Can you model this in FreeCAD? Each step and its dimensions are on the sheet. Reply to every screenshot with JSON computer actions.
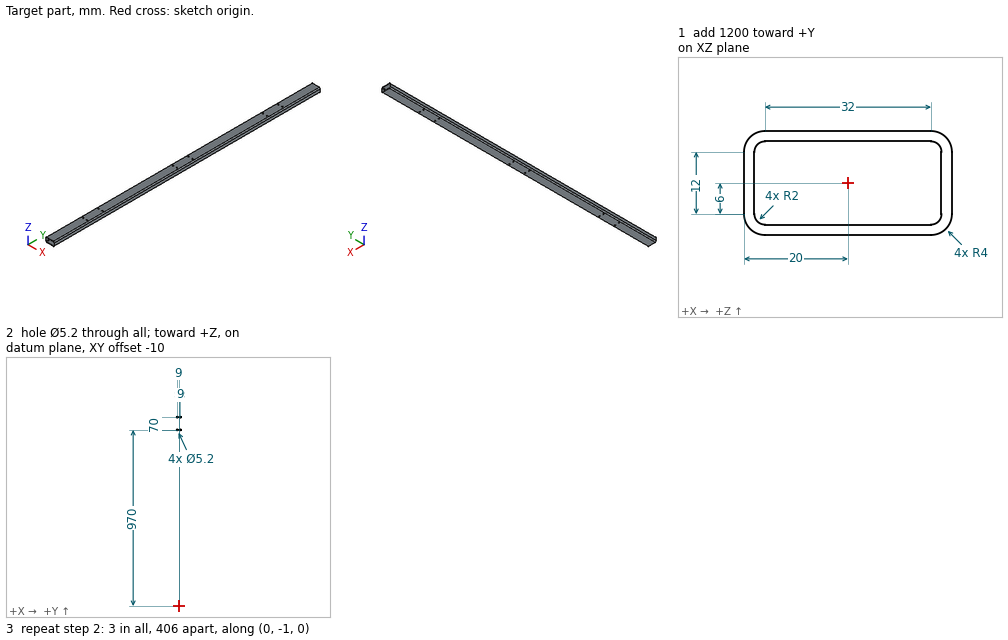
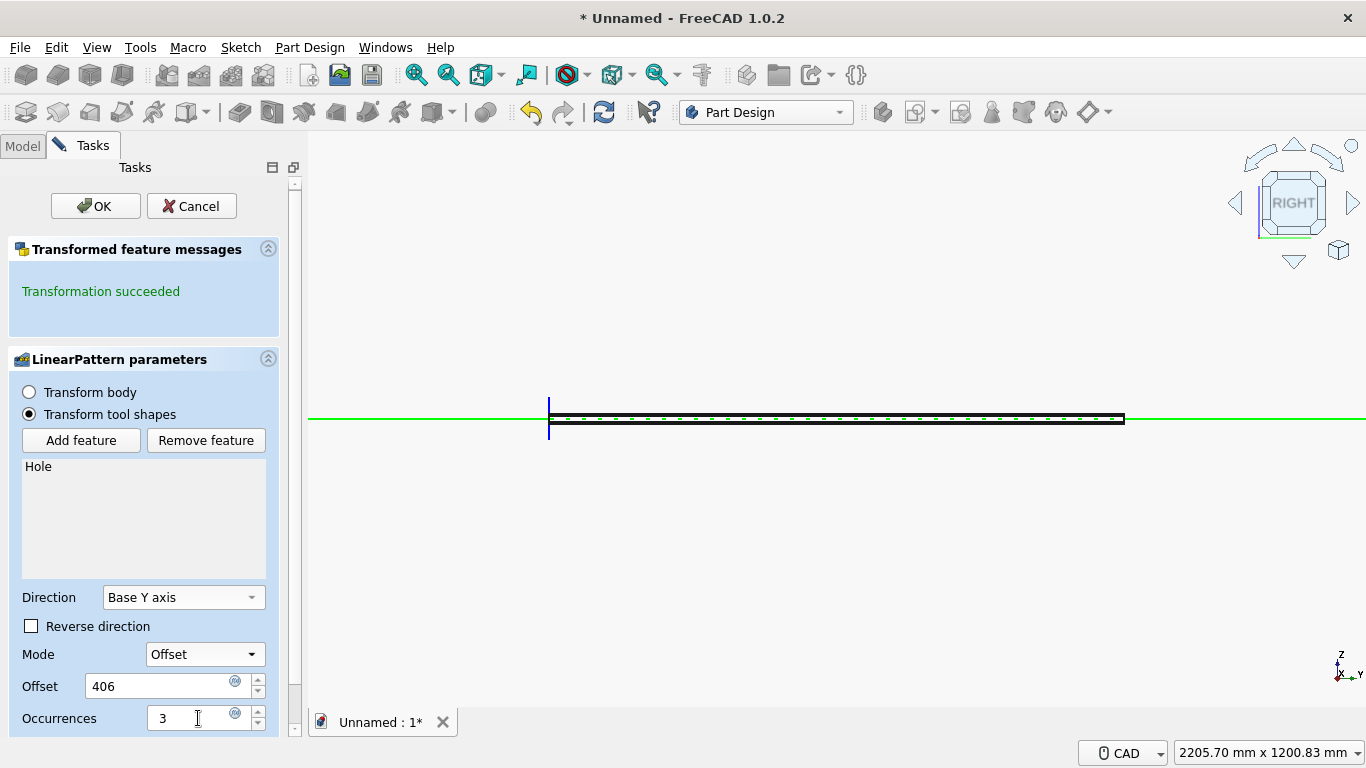
{"action": "left_click", "coordinate": [30, 626]}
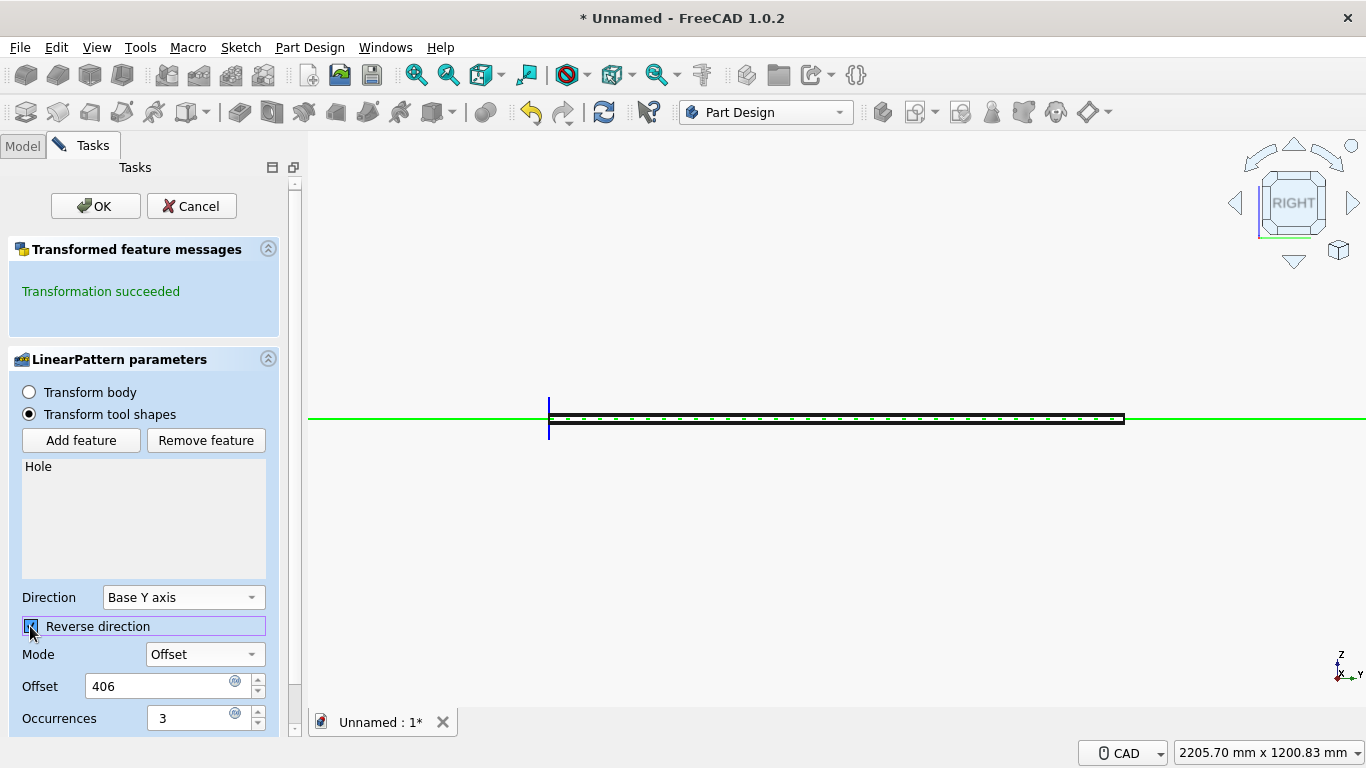
{"action": "left_click", "coordinate": [96, 206]}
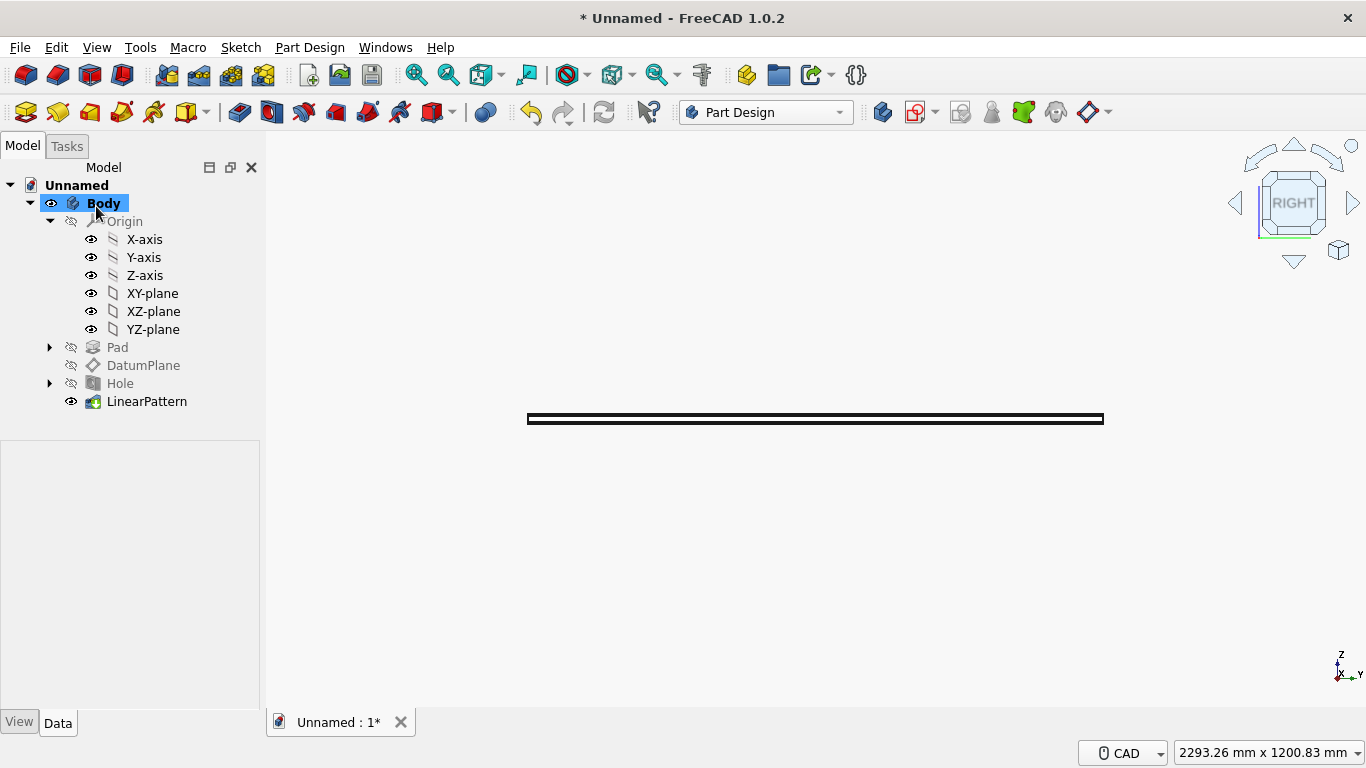
{"action": "key", "text": "0"}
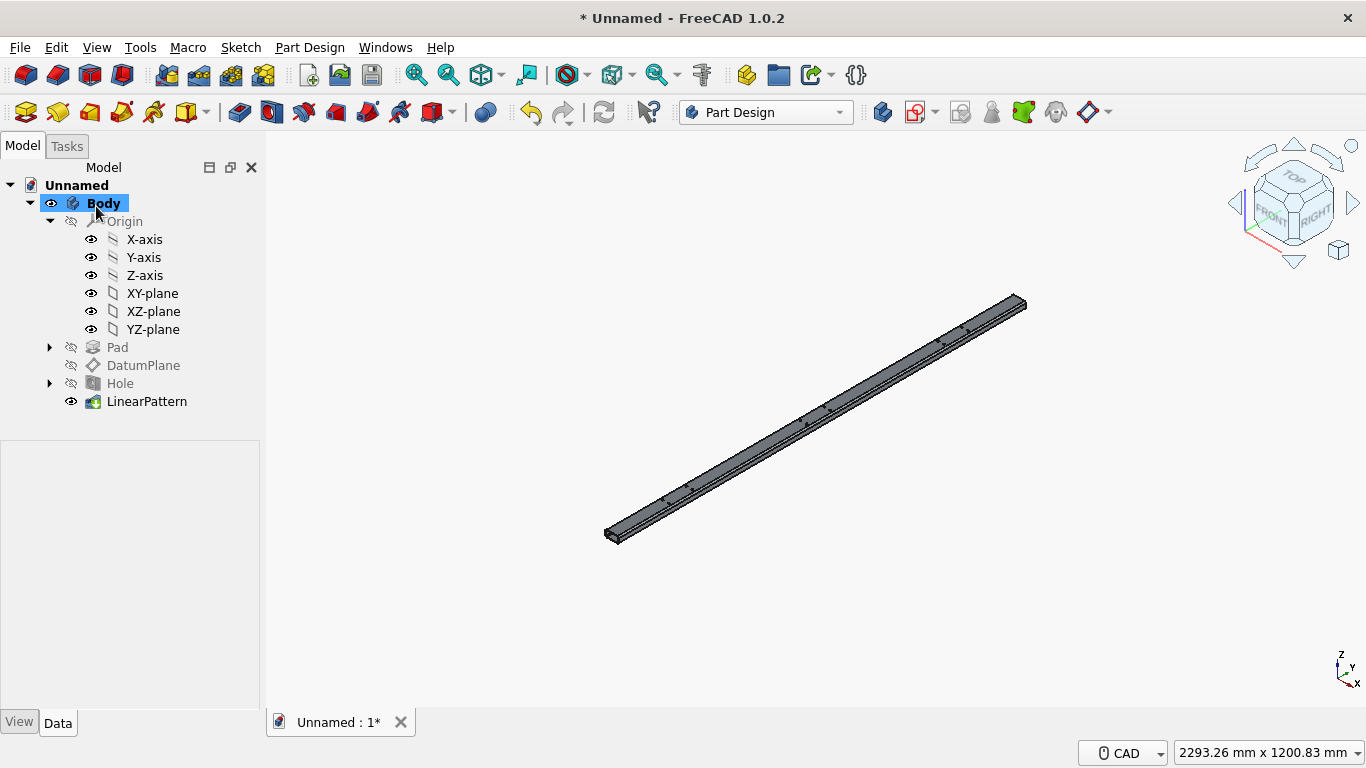
{"action": "left_click", "coordinate": [418, 76]}